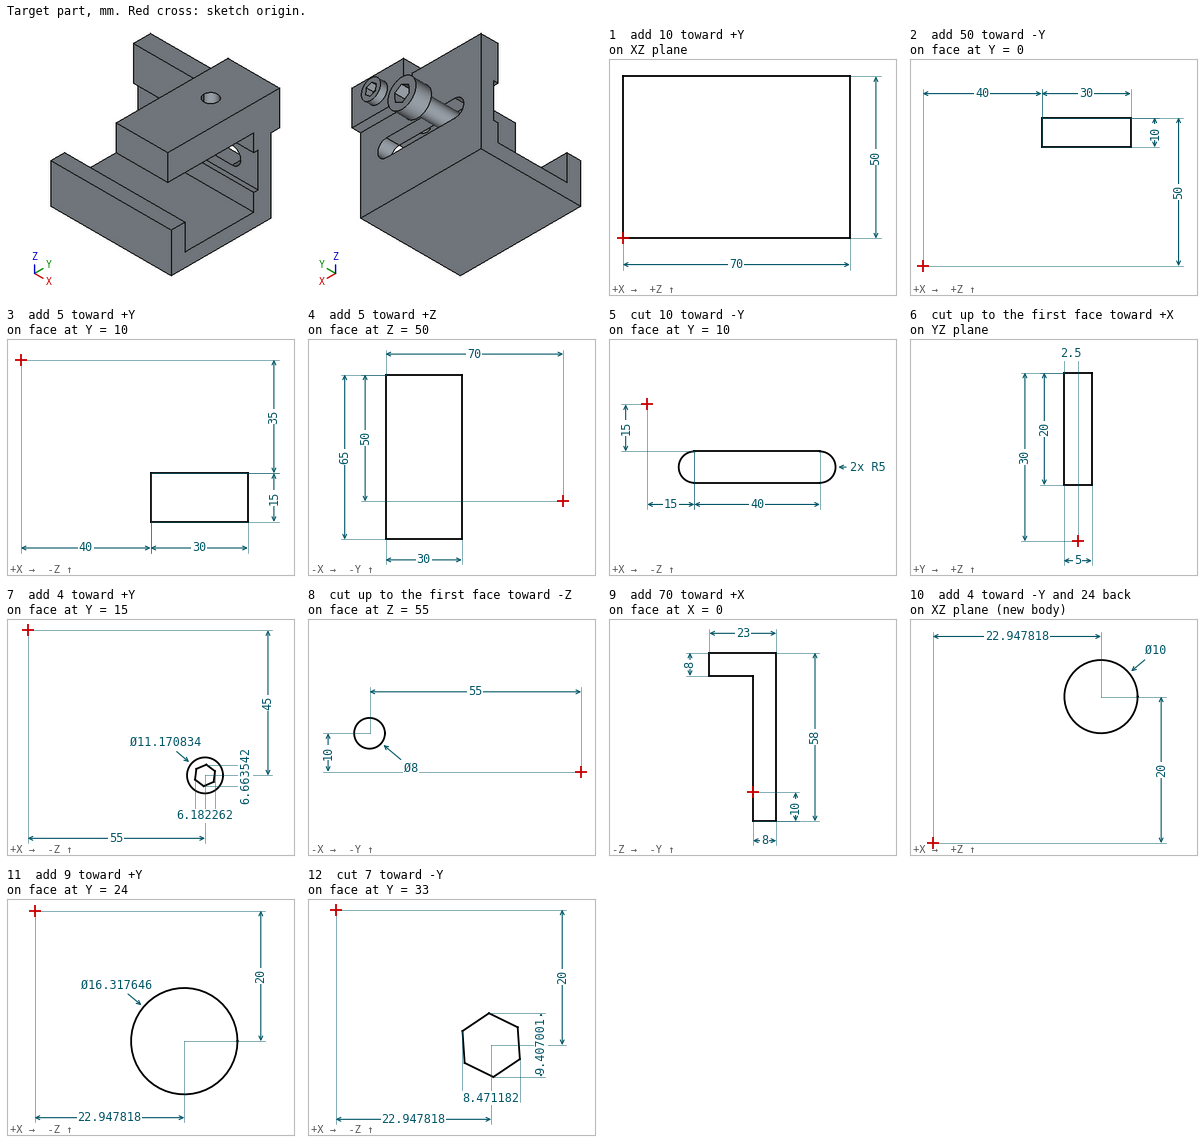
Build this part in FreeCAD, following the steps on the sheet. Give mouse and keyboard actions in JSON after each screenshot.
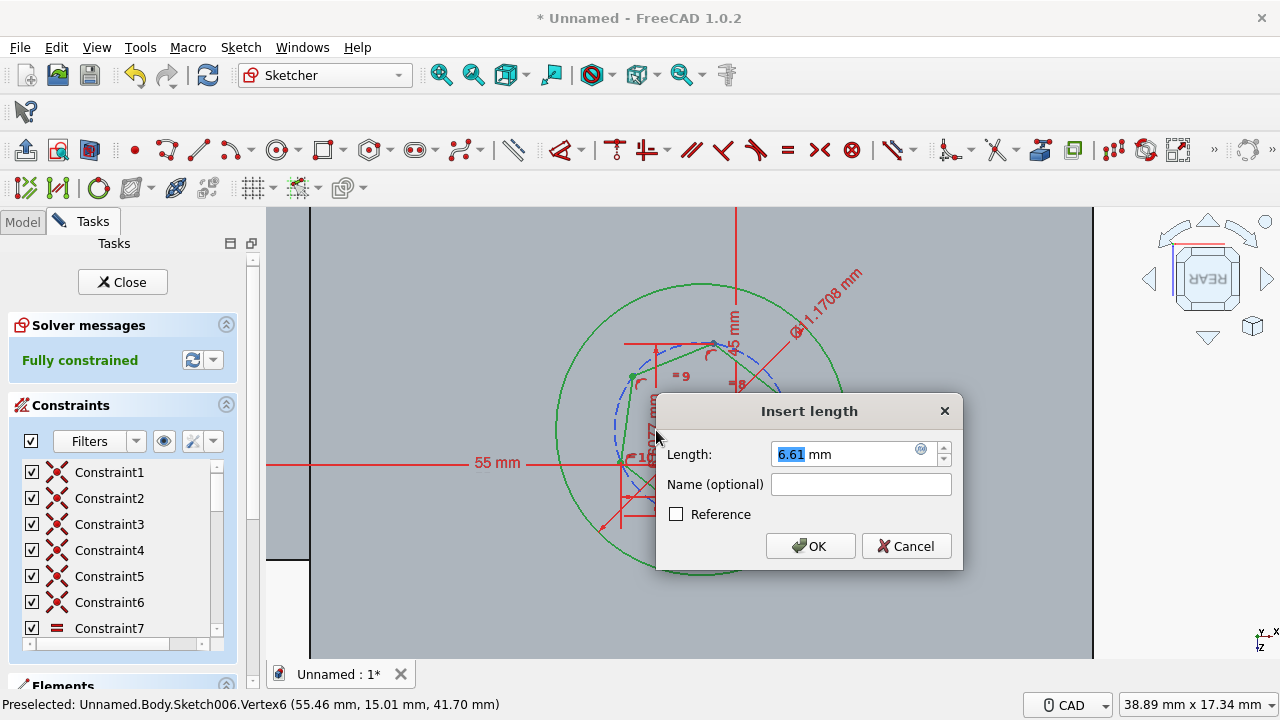
{"action": "type", "text": "6.663542"}
{"action": "key", "text": "Return"}
{"action": "key", "text": "Escape"}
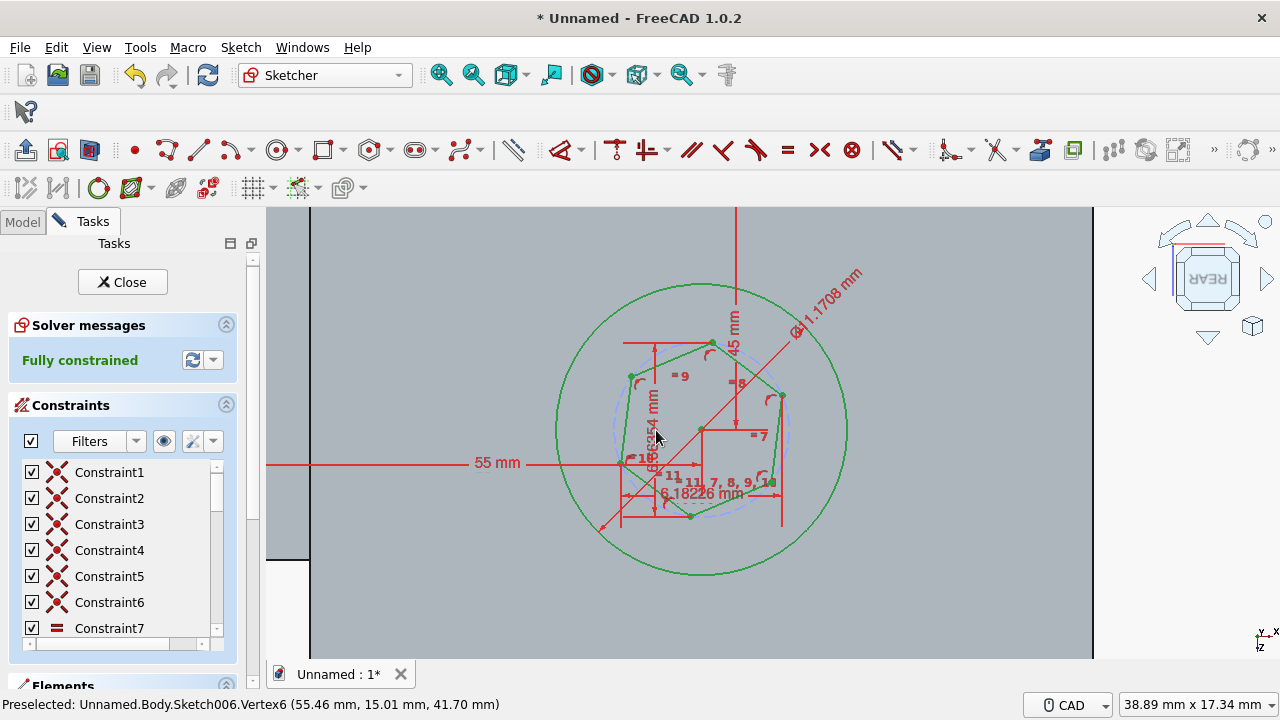
{"action": "left_click", "coordinate": [123, 282]}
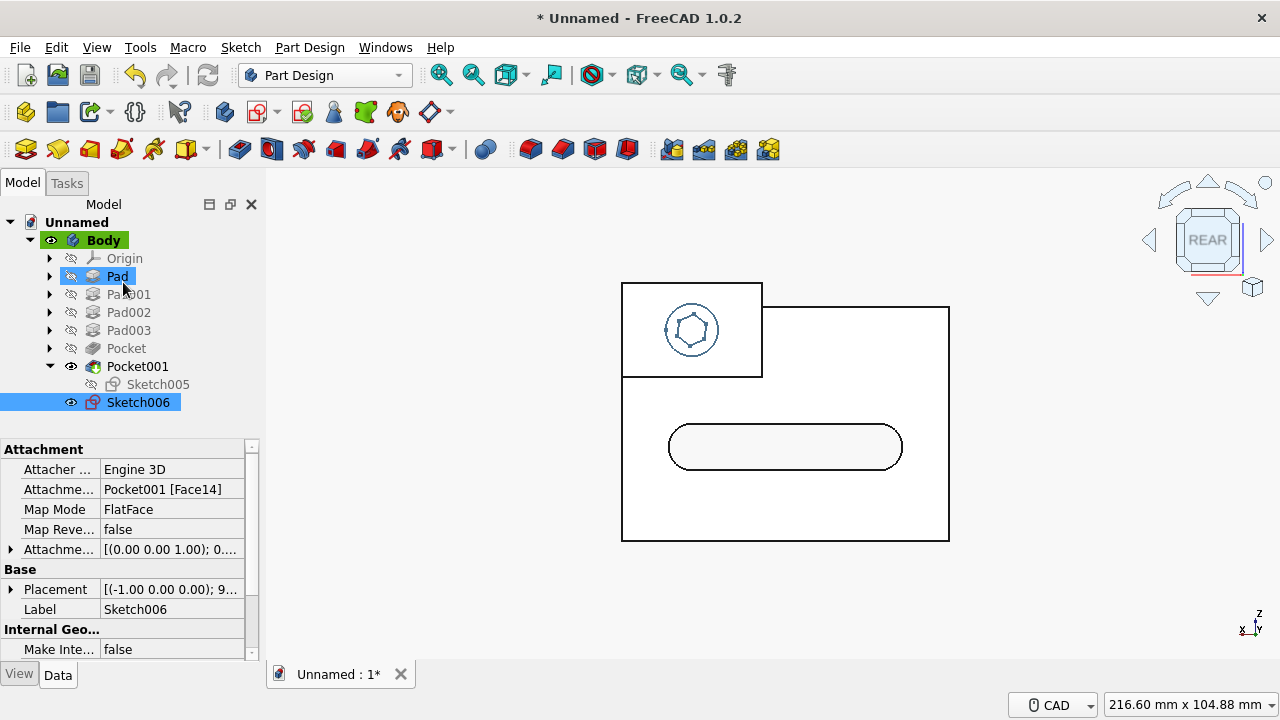
{"action": "left_click", "coordinate": [26, 150]}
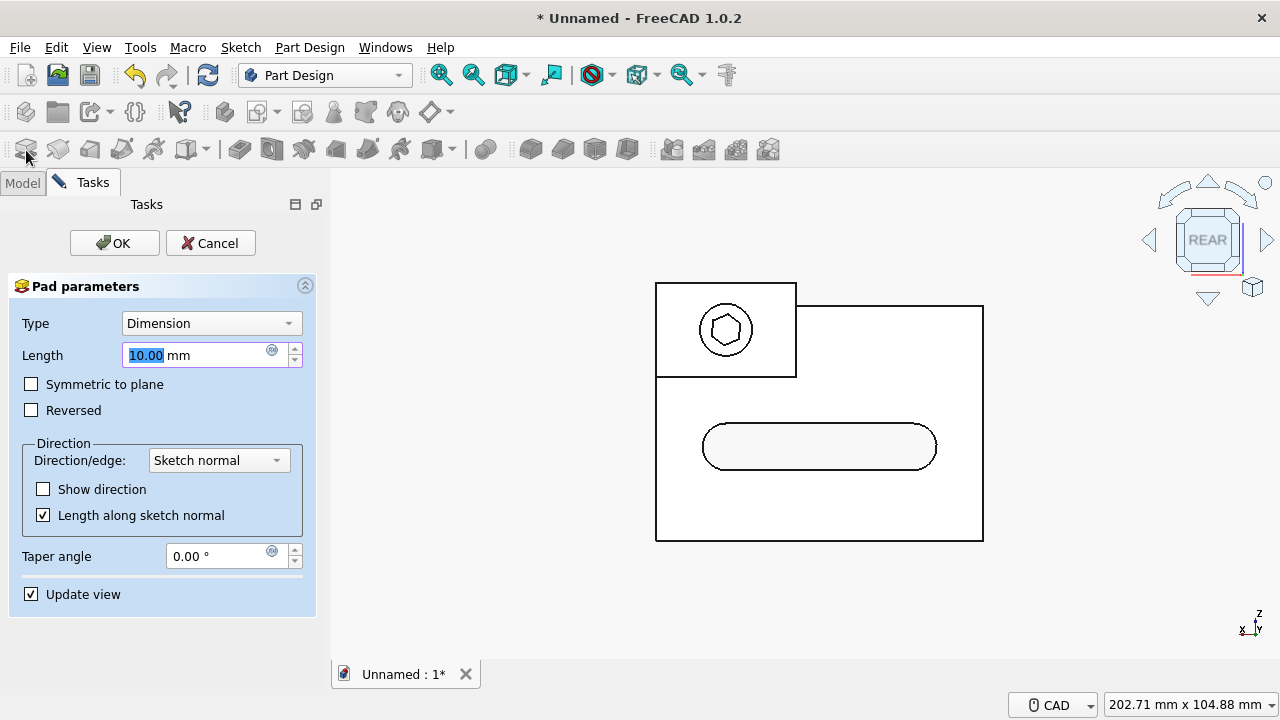
{"action": "type", "text": "4"}
{"action": "key", "text": "Tab"}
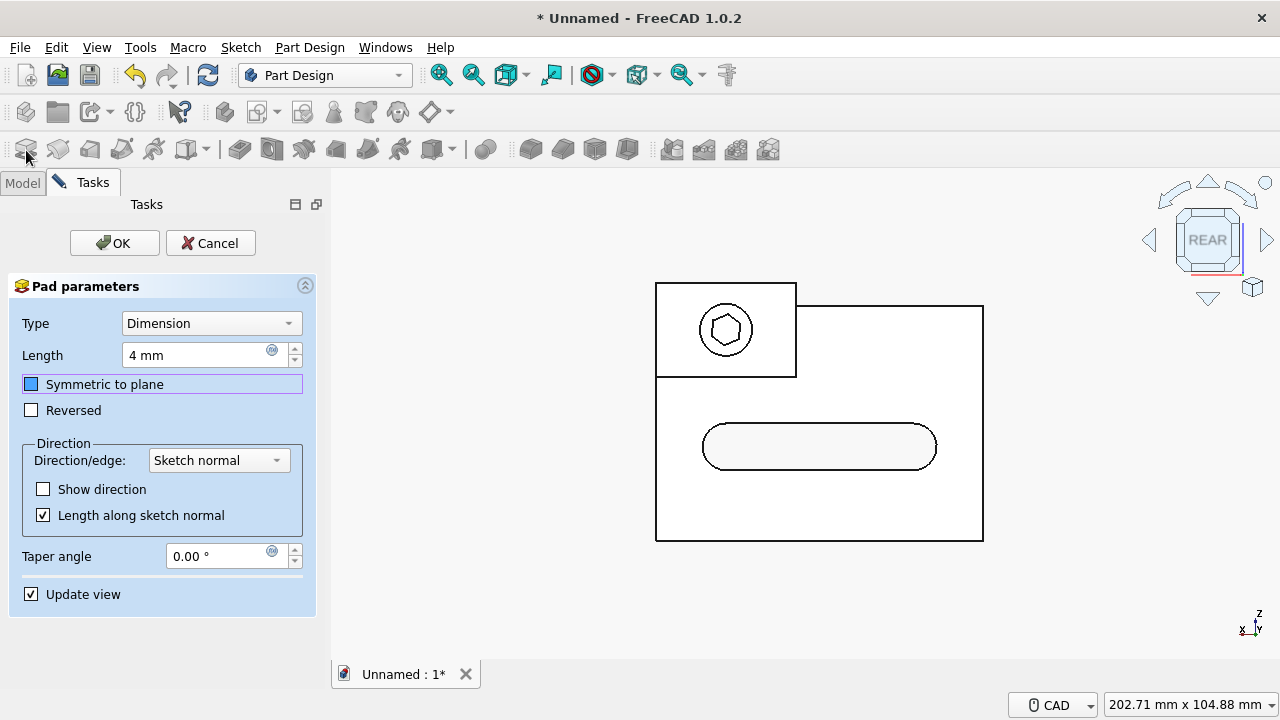
{"action": "left_click", "coordinate": [115, 243]}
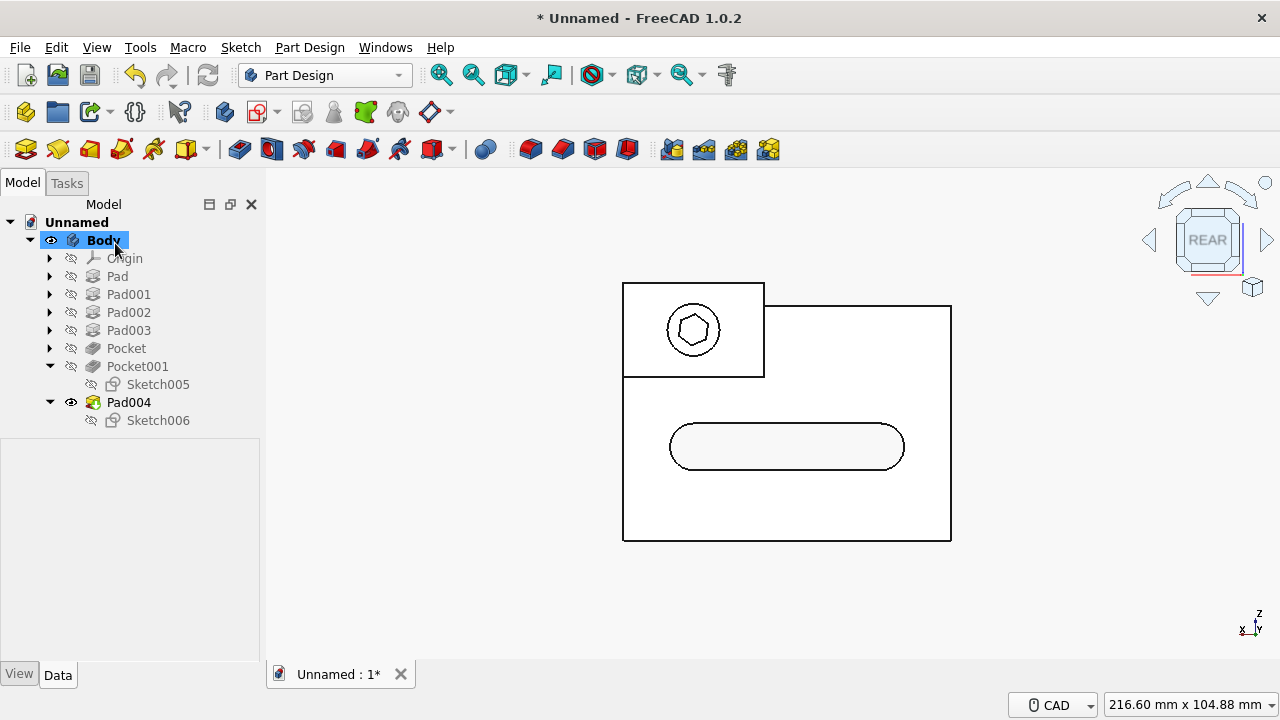
{"action": "key", "text": "0"}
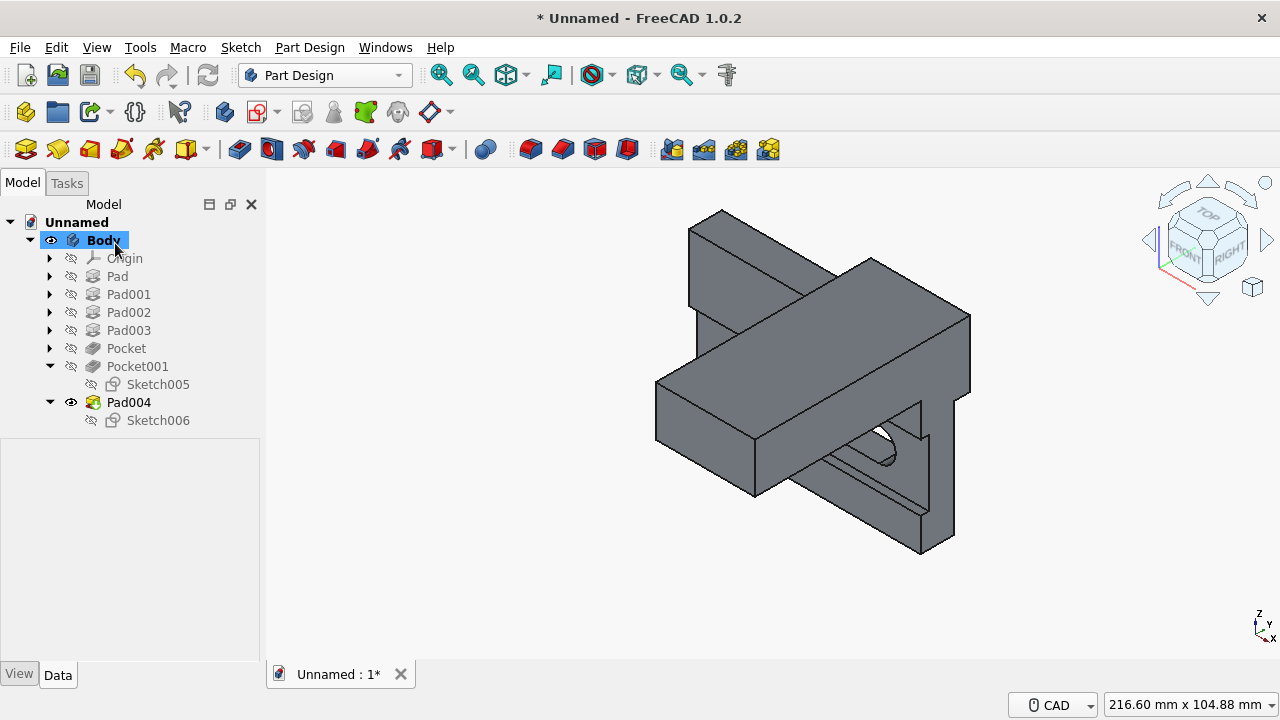
{"action": "left_click", "coordinate": [844, 330]}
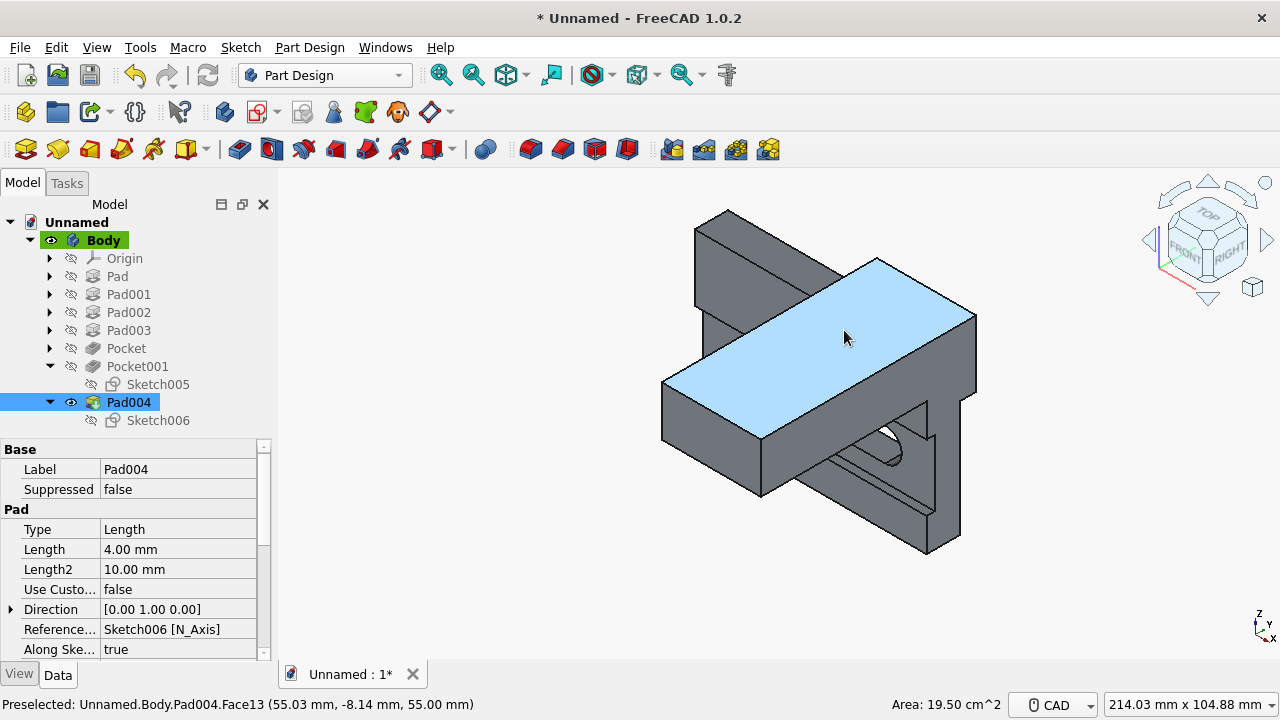
{"action": "left_click", "coordinate": [258, 112]}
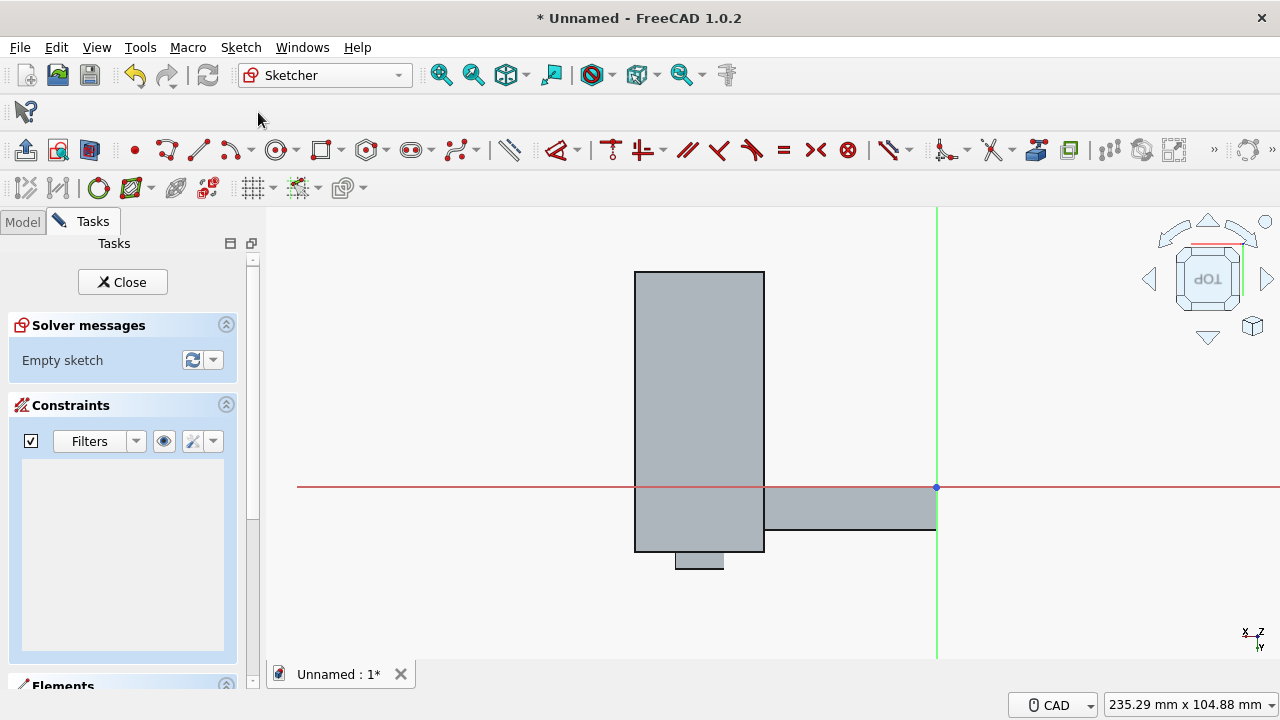
{"action": "scroll", "coordinate": [699, 446], "scroll_direction": "up", "scroll_amount": 10}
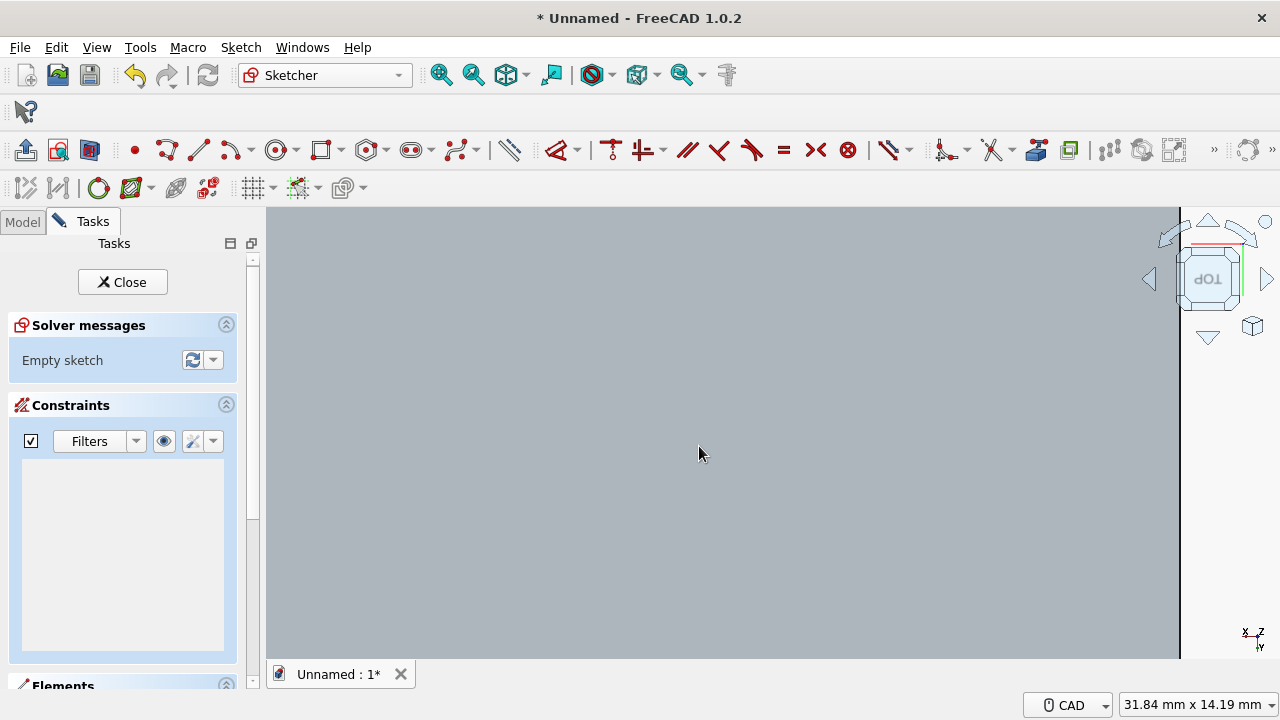
{"action": "left_click", "coordinate": [276, 150]}